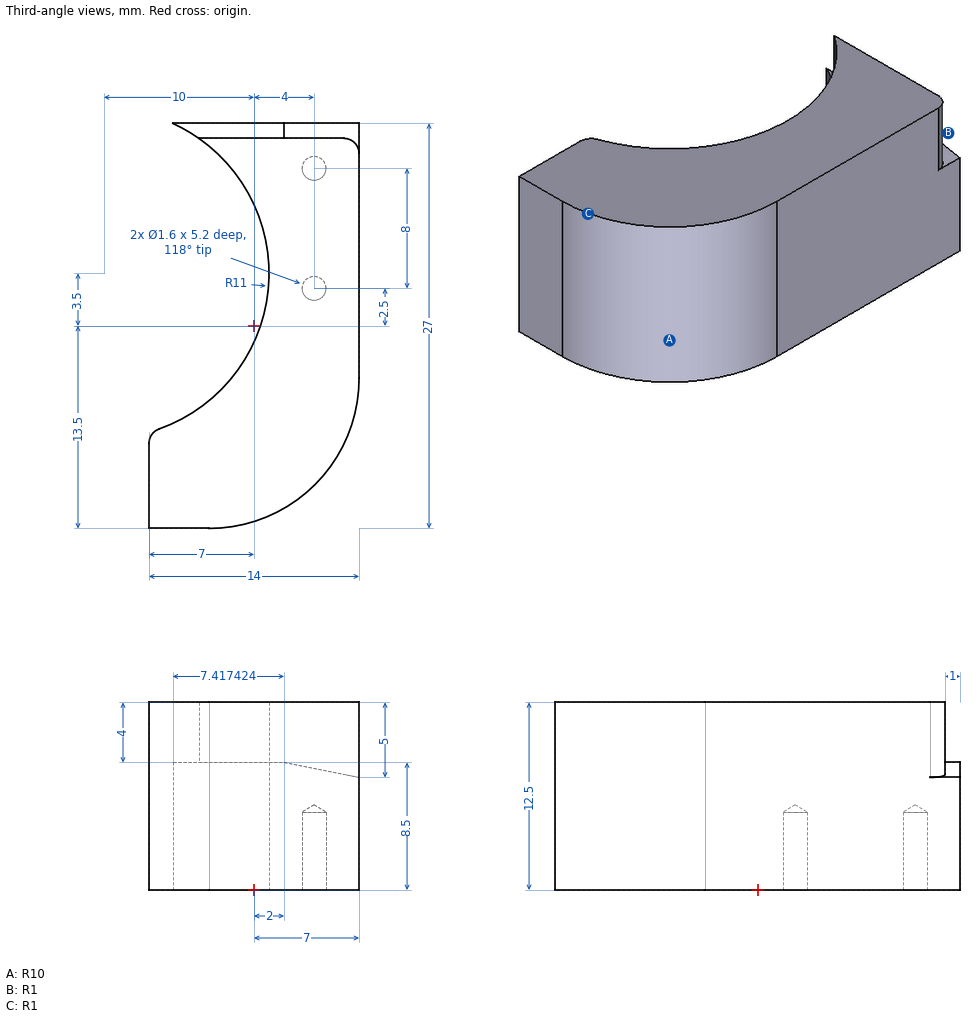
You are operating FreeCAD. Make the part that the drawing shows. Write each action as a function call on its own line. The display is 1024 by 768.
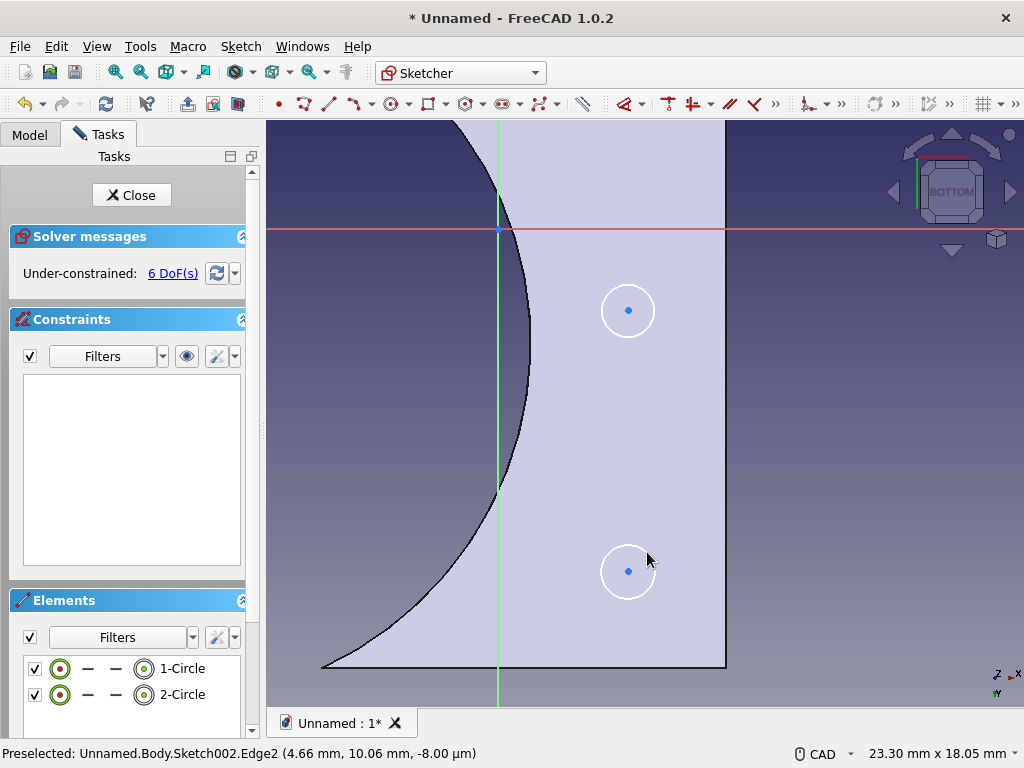
click(646, 292)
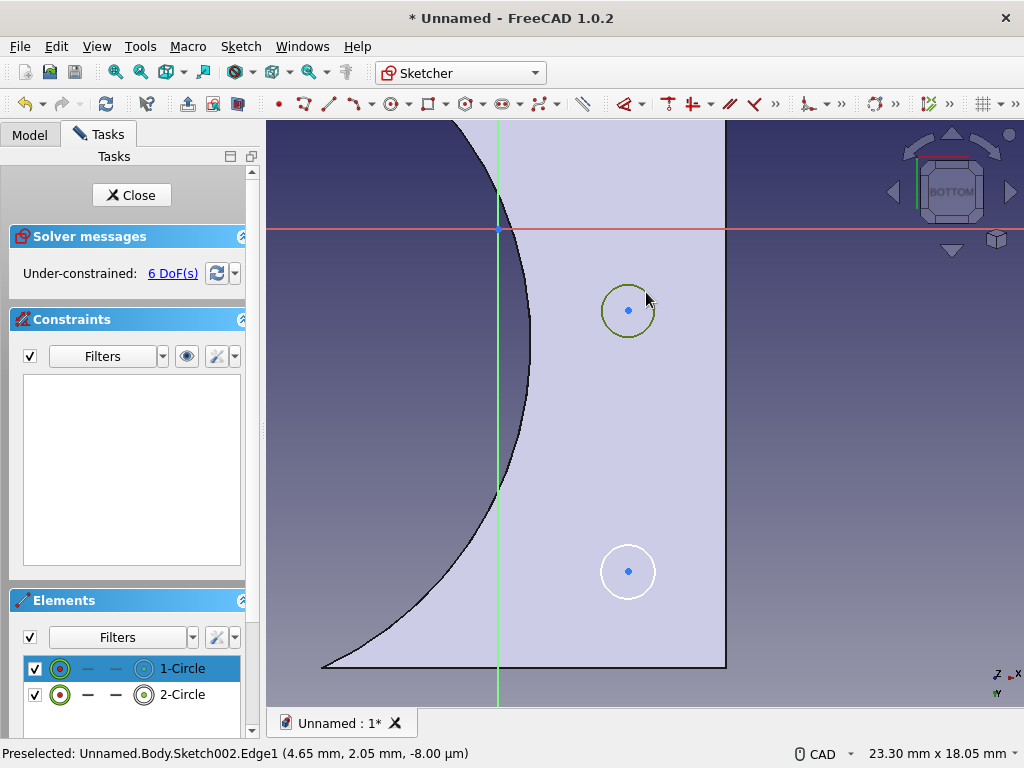
click(647, 553)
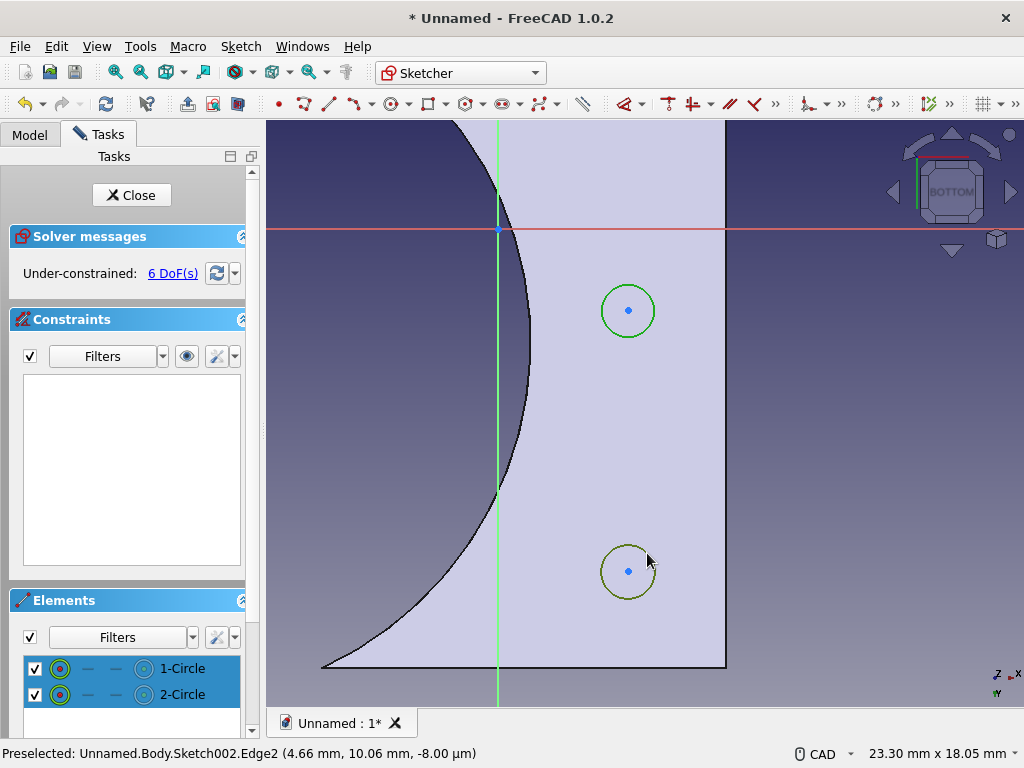
key(e)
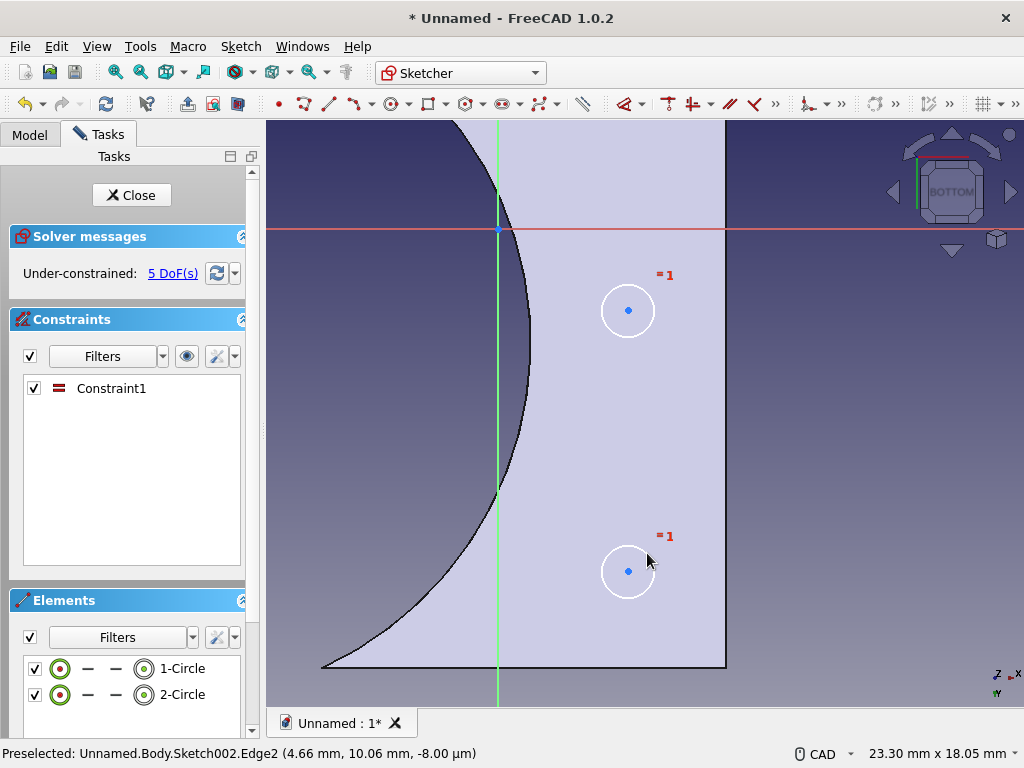
click(628, 311)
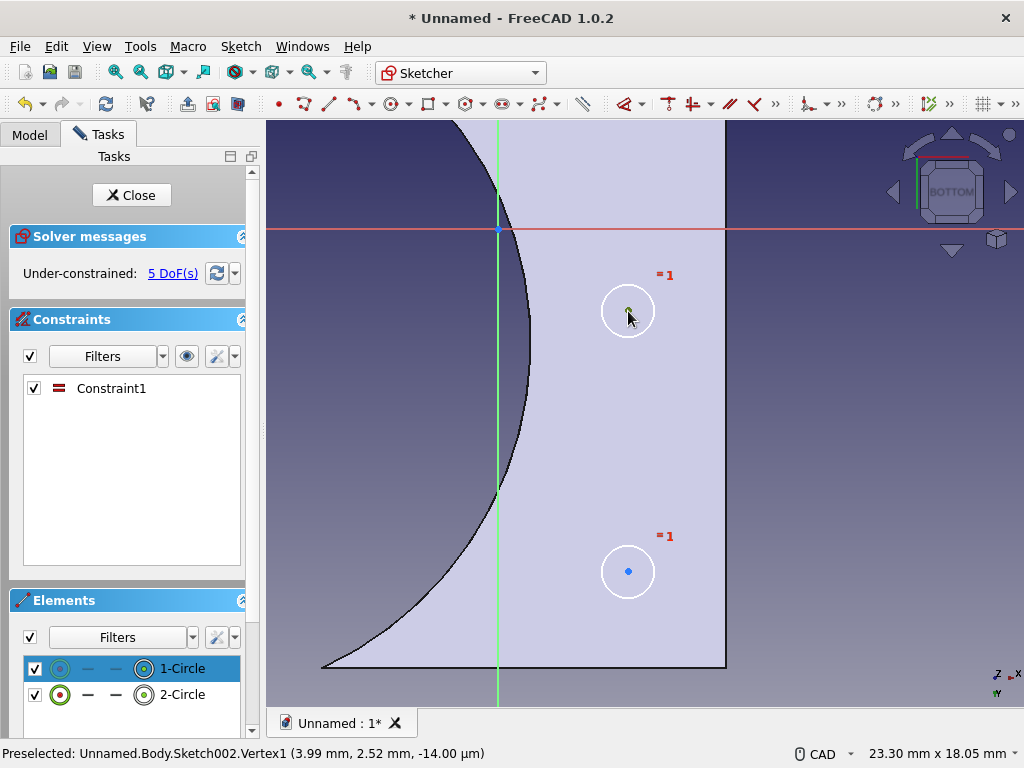
click(628, 572)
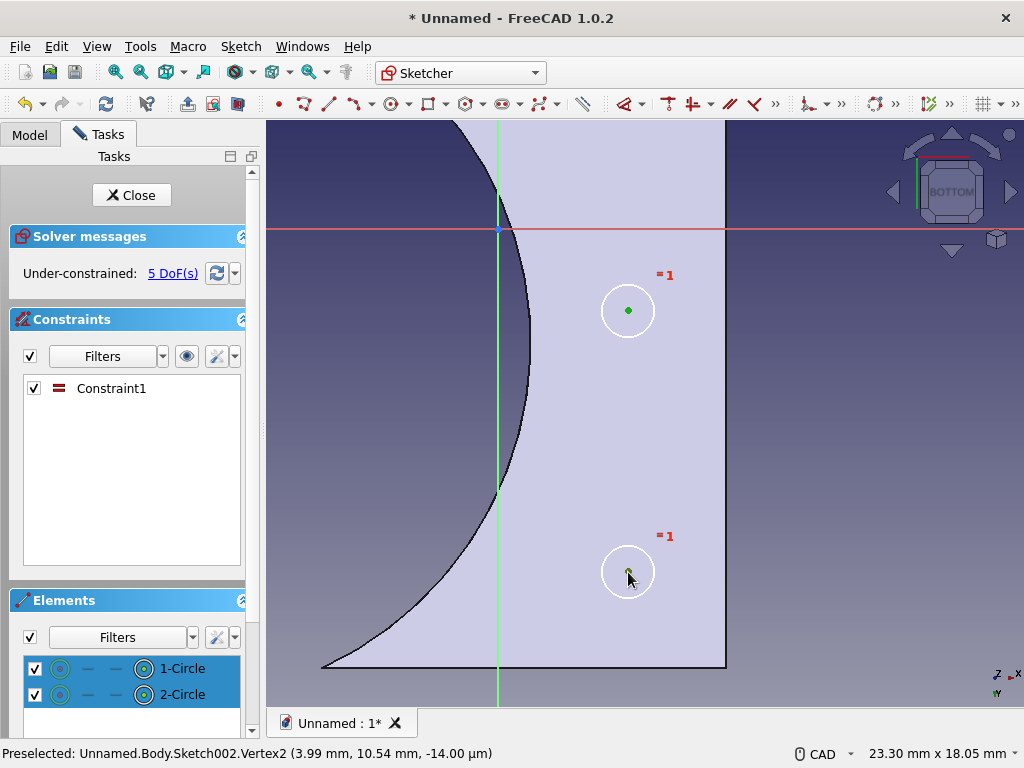
click(710, 104)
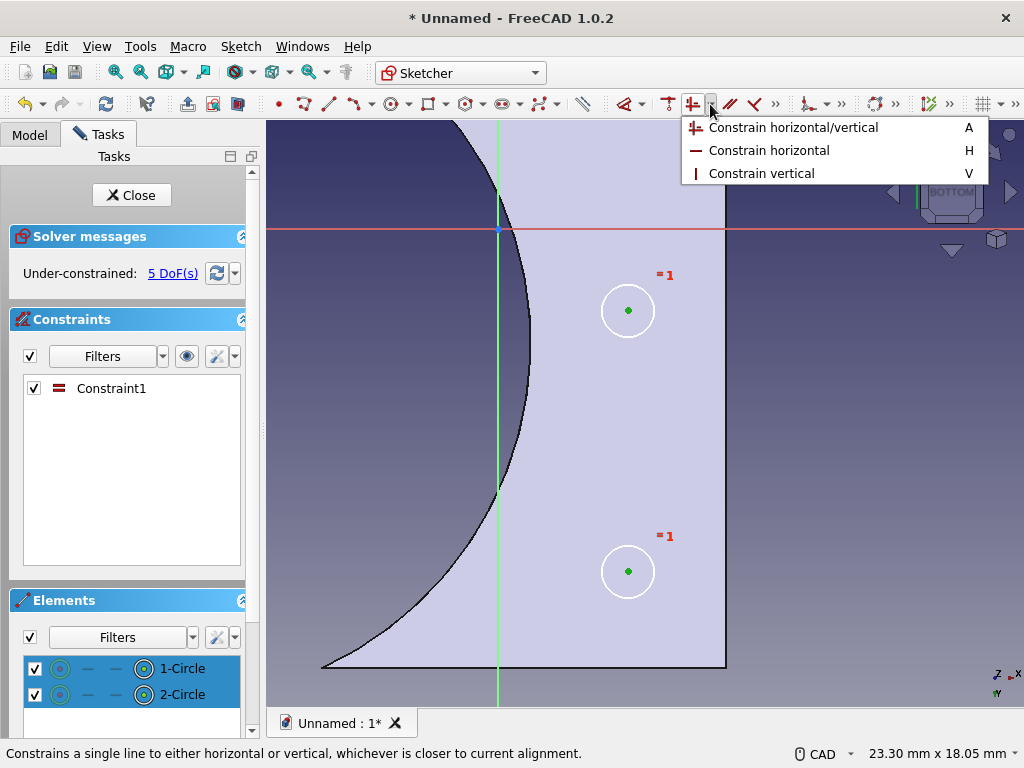
click(835, 174)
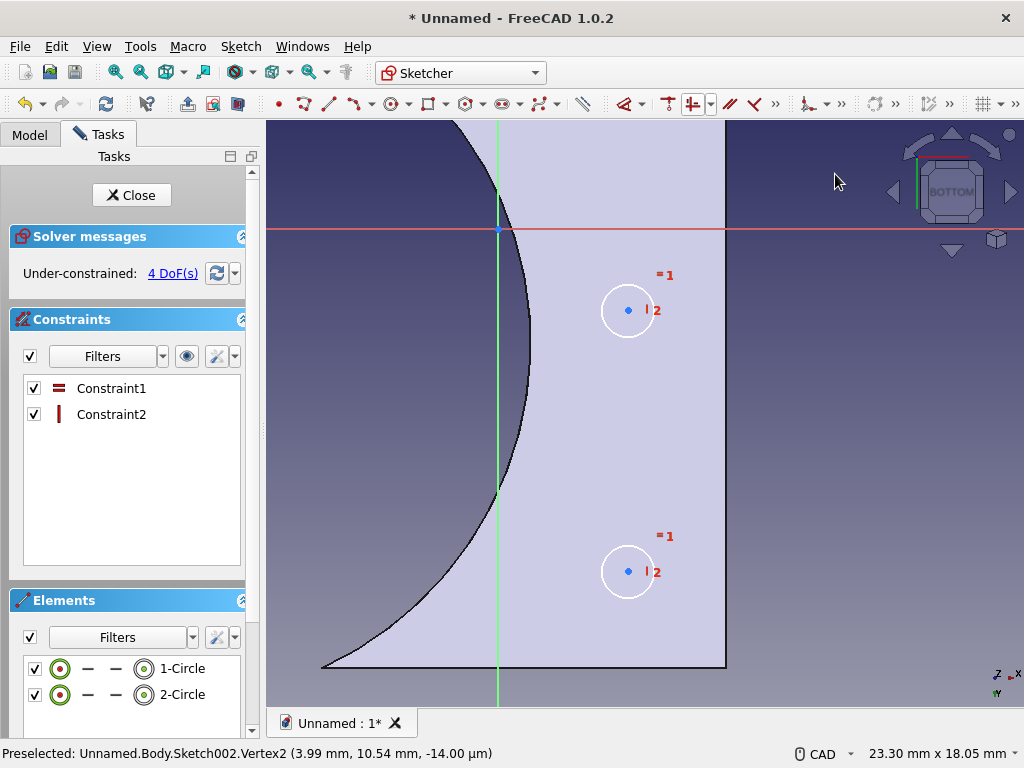
click(624, 104)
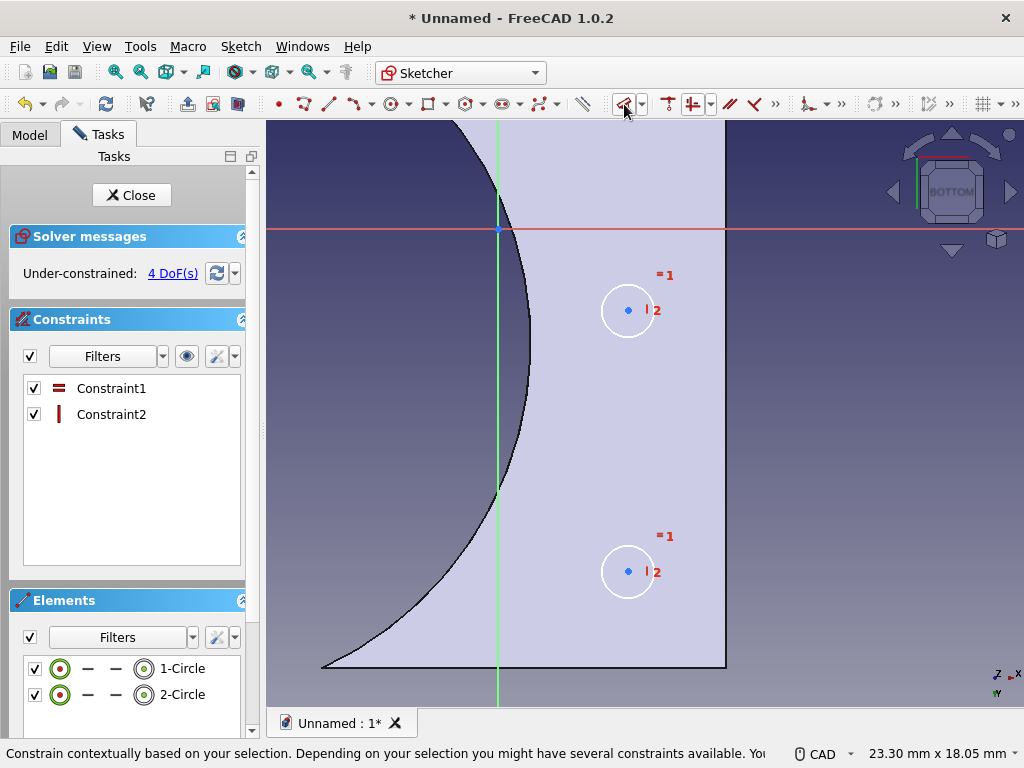
click(646, 292)
click(668, 269)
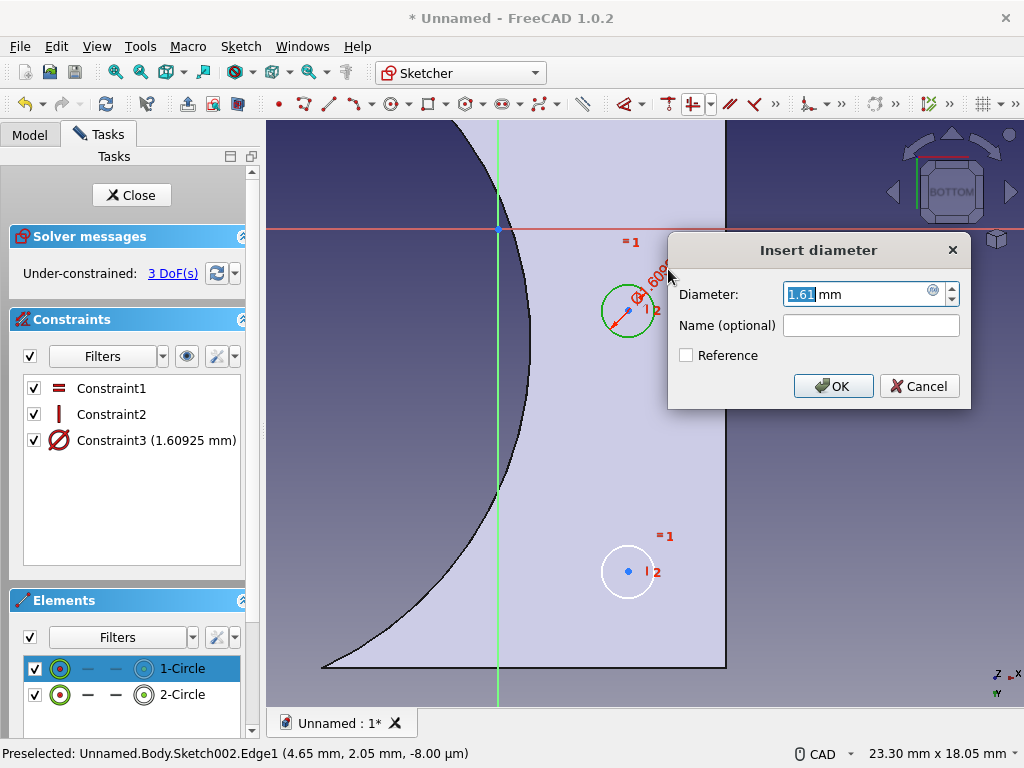
text(1.6)
key(Return)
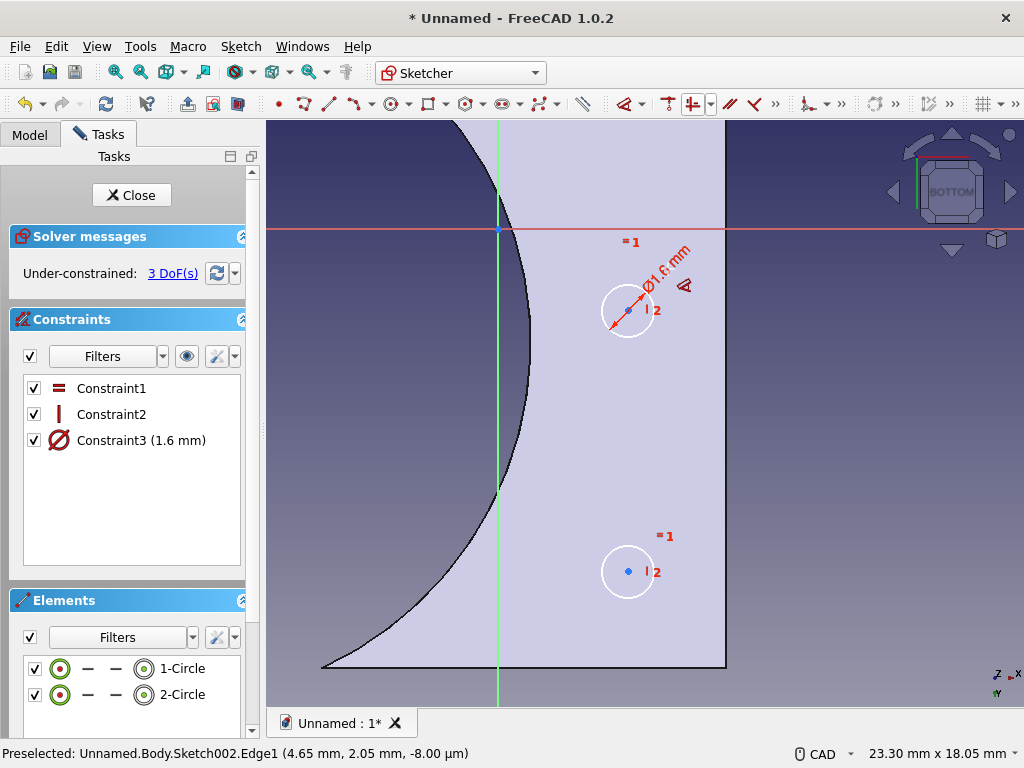
click(628, 311)
click(563, 195)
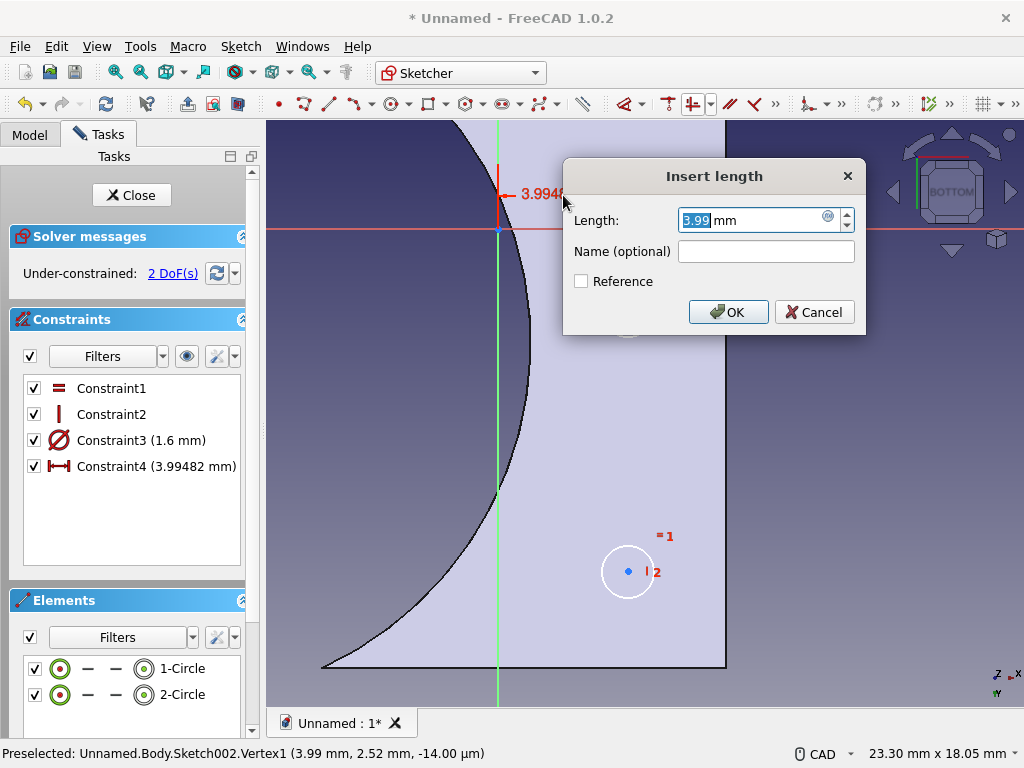
text(4)
key(Return)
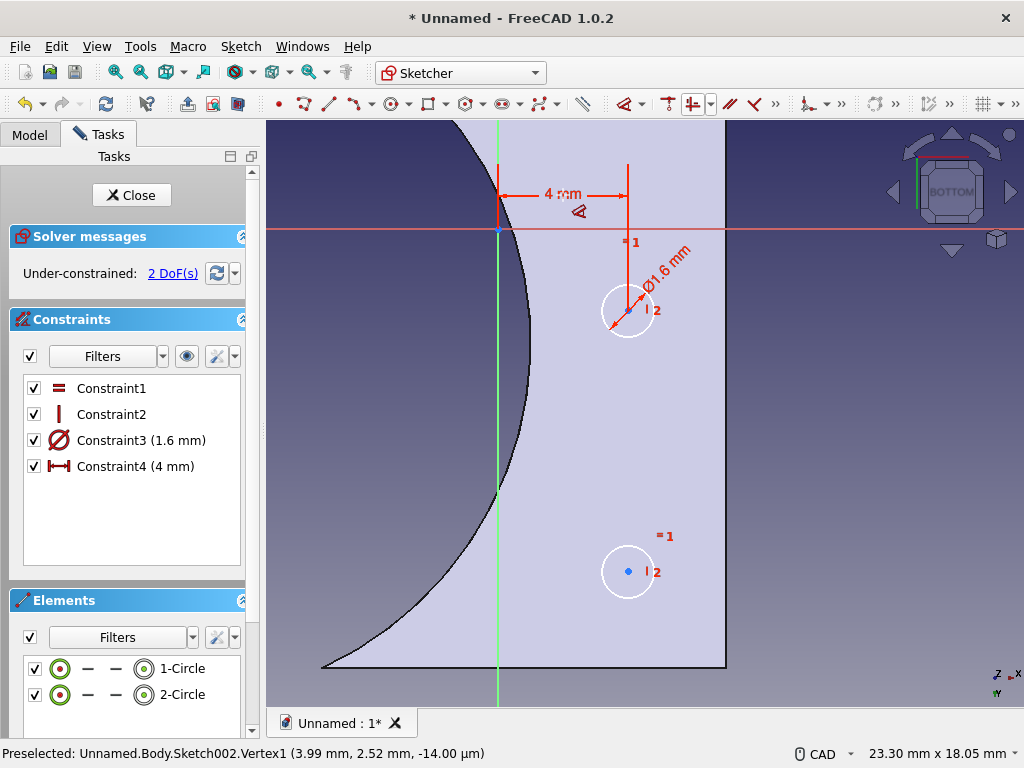
click(628, 311)